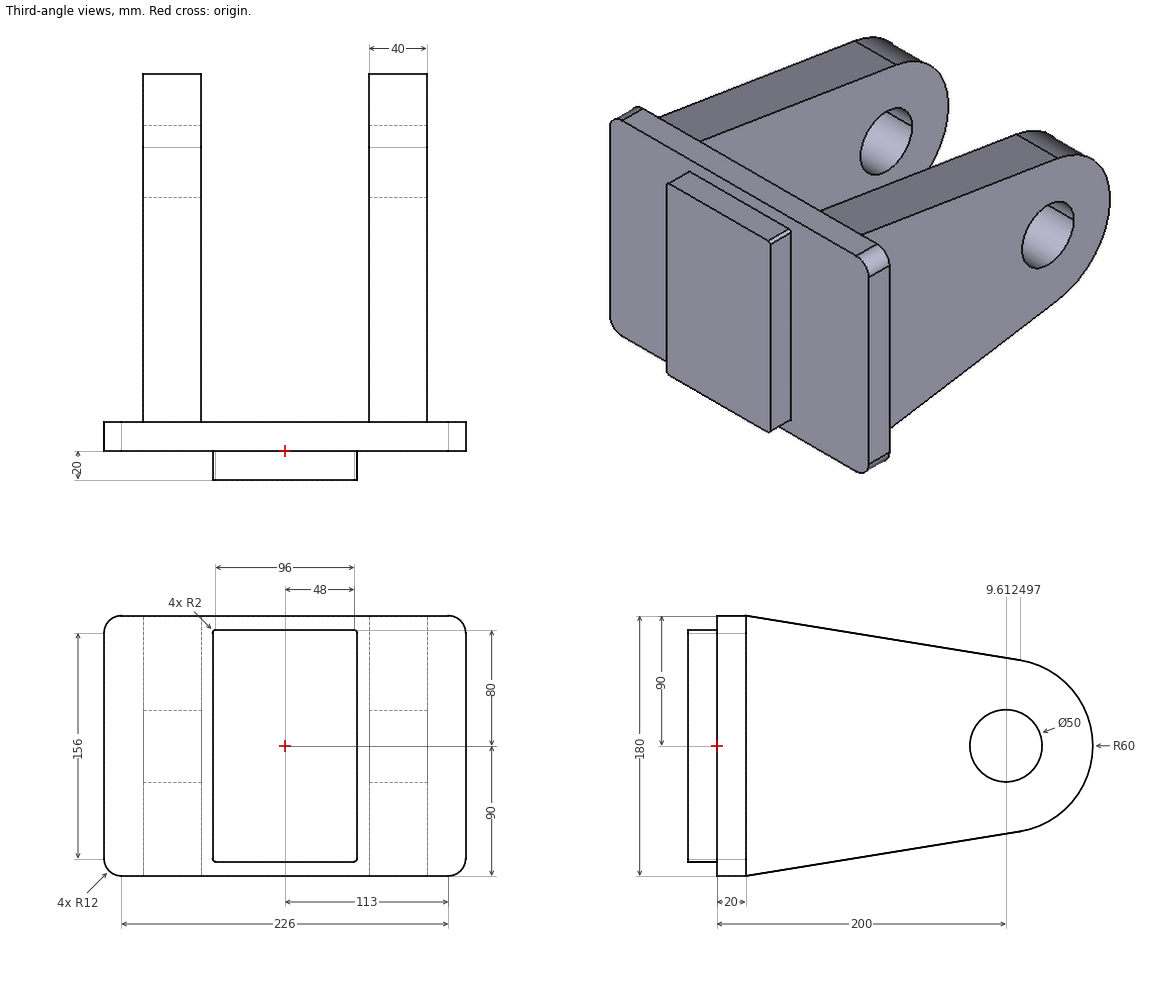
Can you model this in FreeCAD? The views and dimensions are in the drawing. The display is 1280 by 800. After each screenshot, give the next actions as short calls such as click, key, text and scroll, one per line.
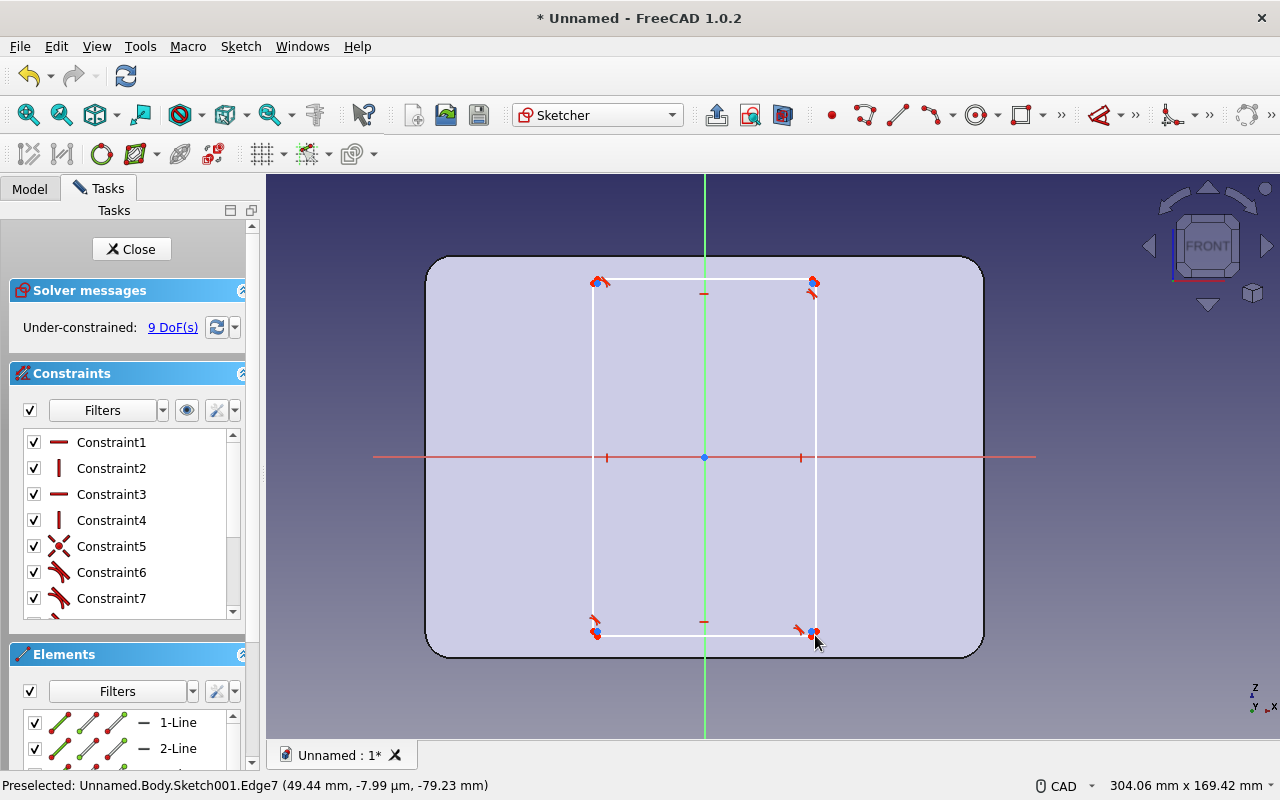
click(816, 562)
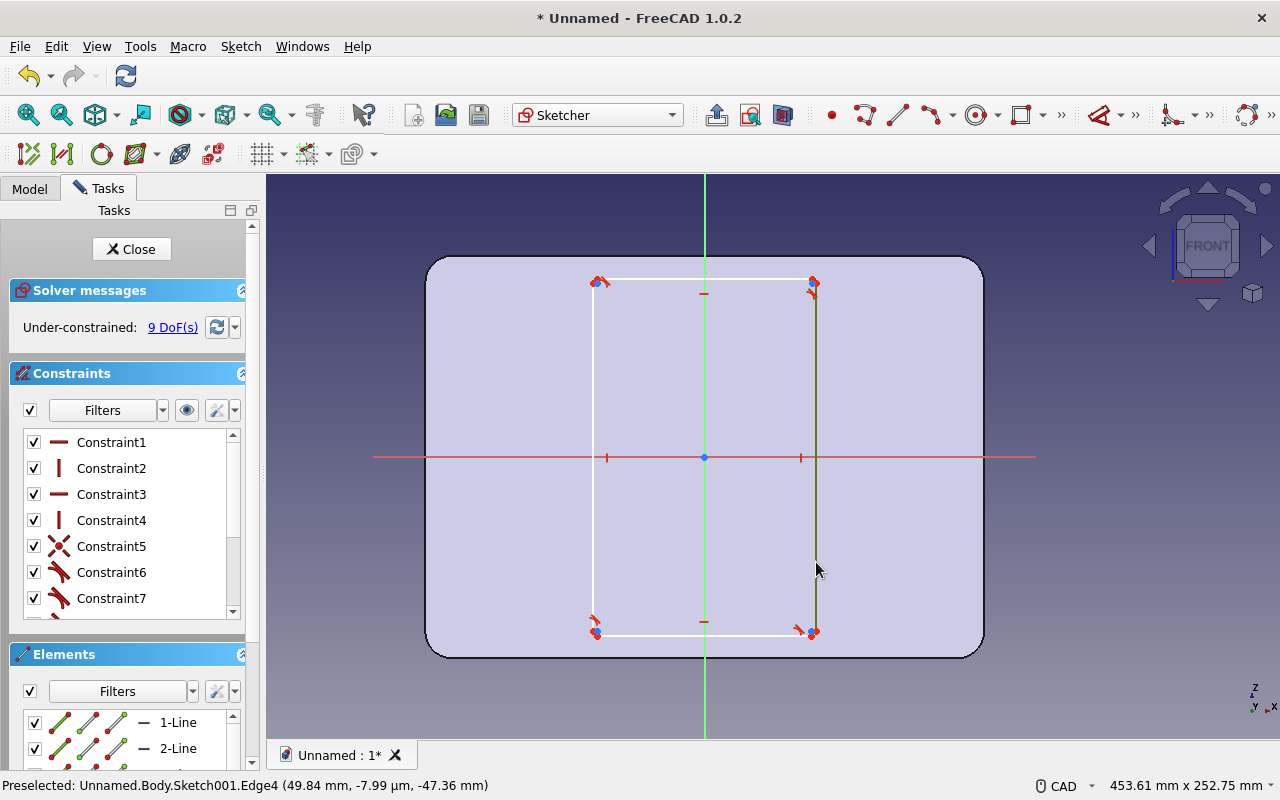
scroll(815, 281, up, 8)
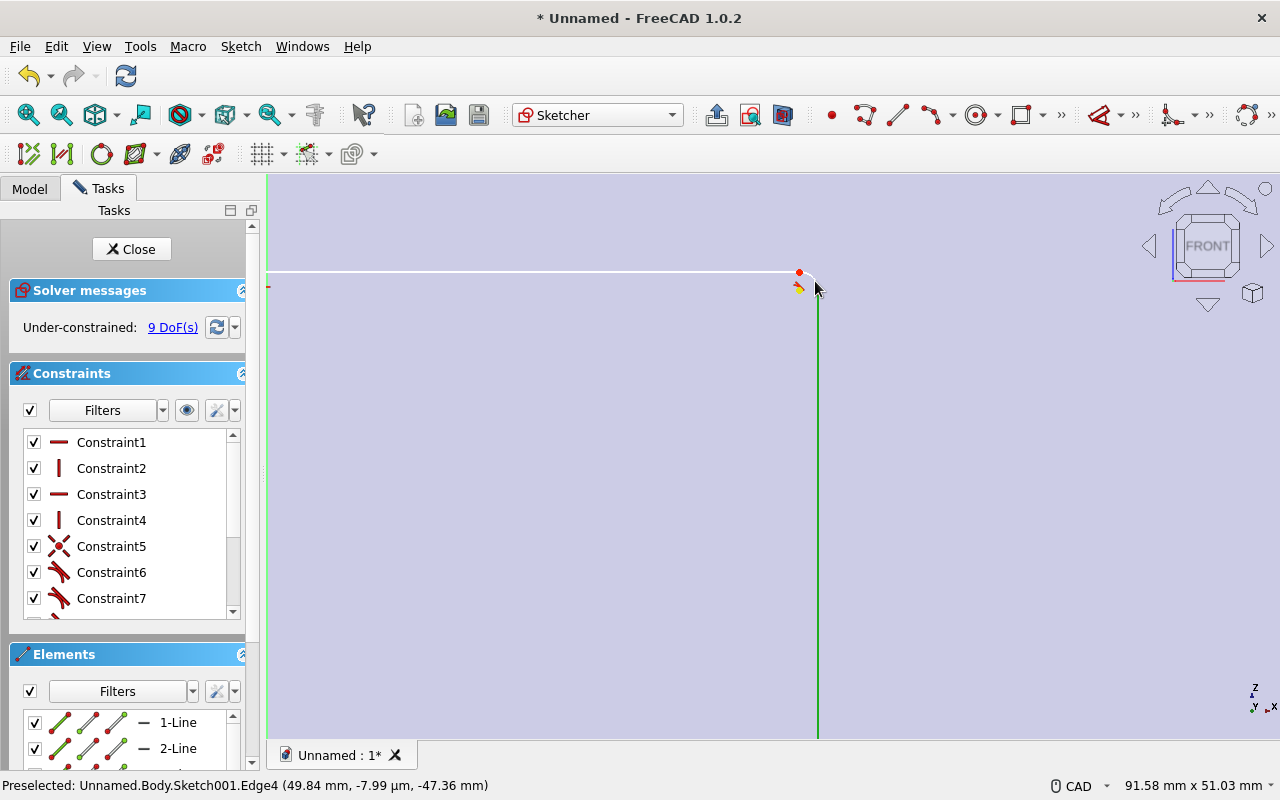
click(813, 278)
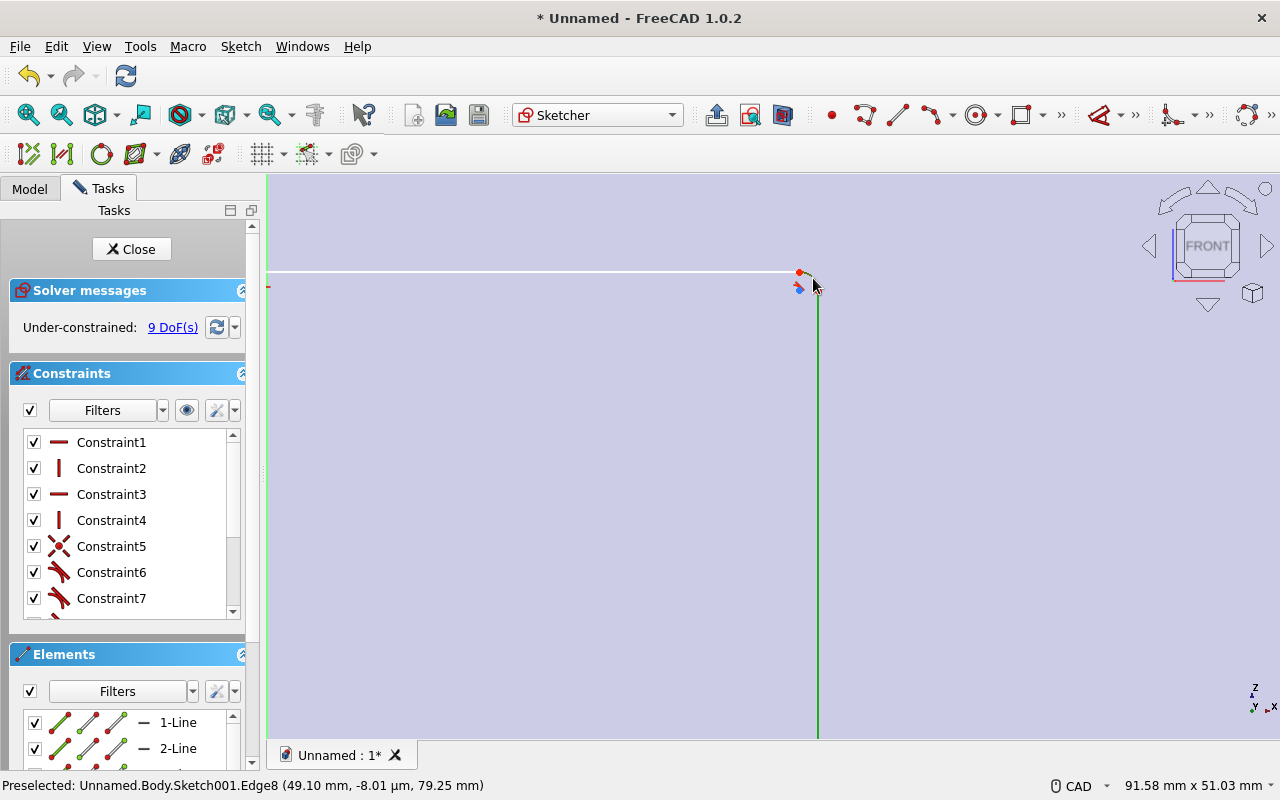
key(t)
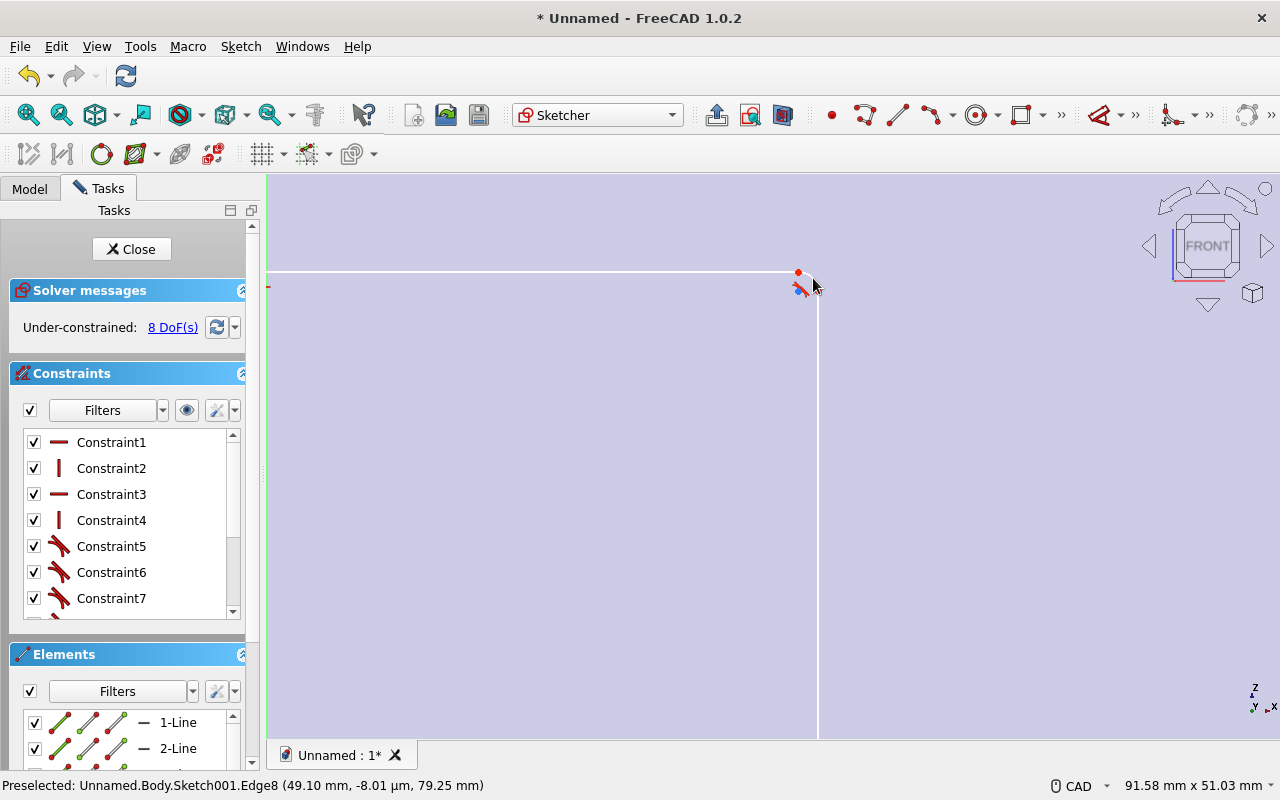
scroll(815, 280, down, 8)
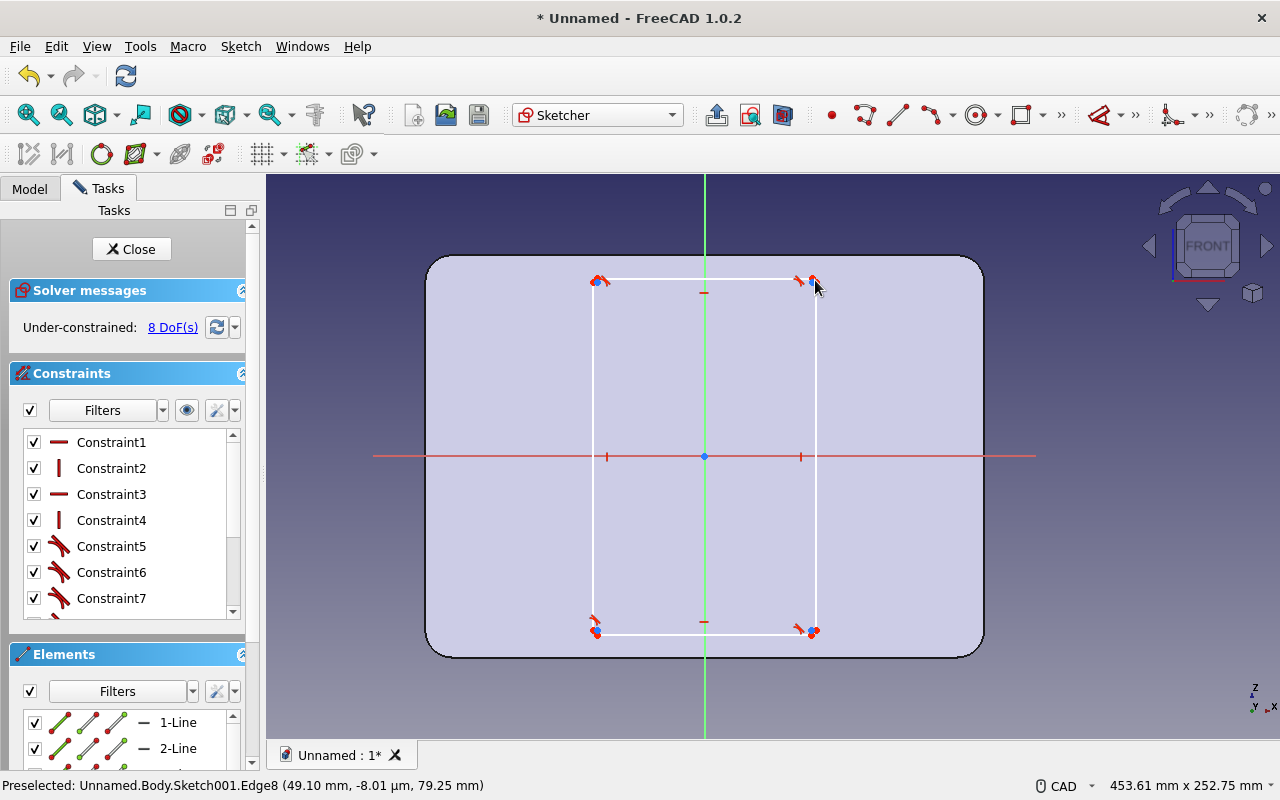
scroll(595, 279, up, 11)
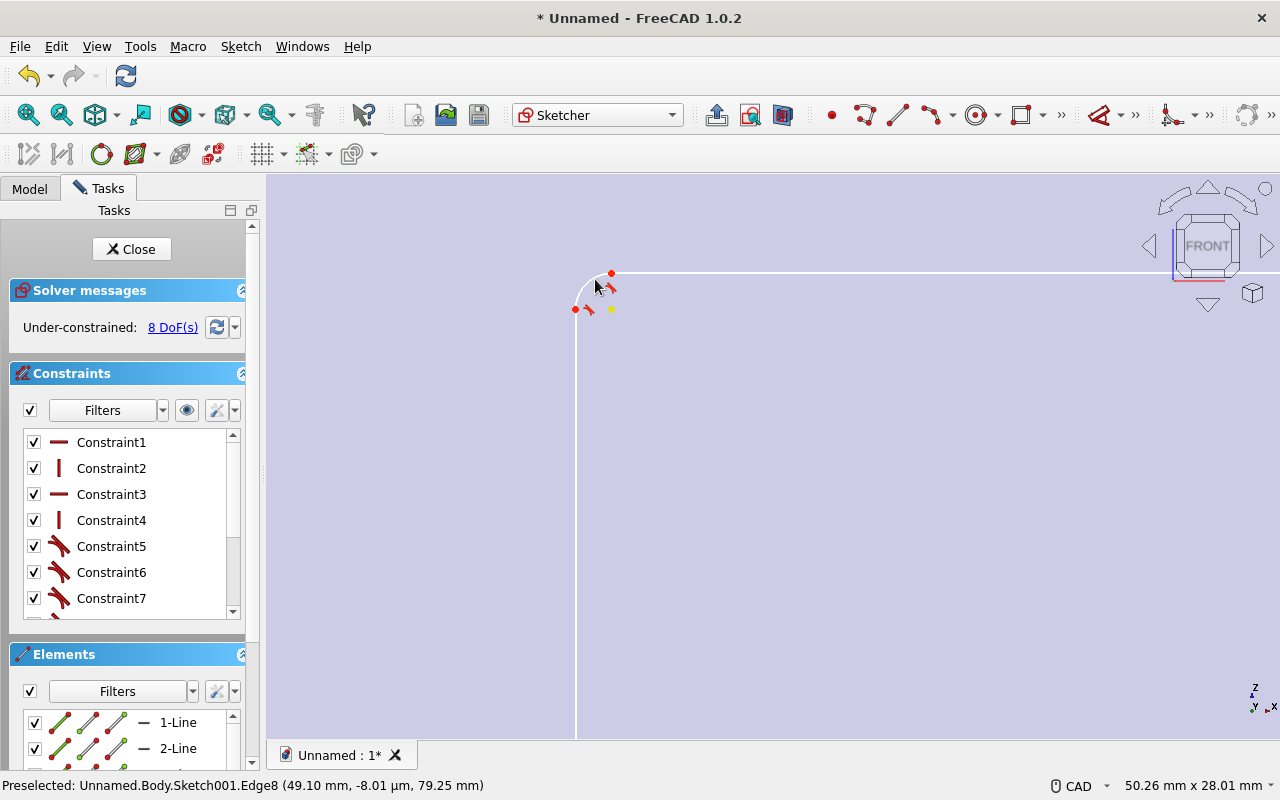
click(595, 277)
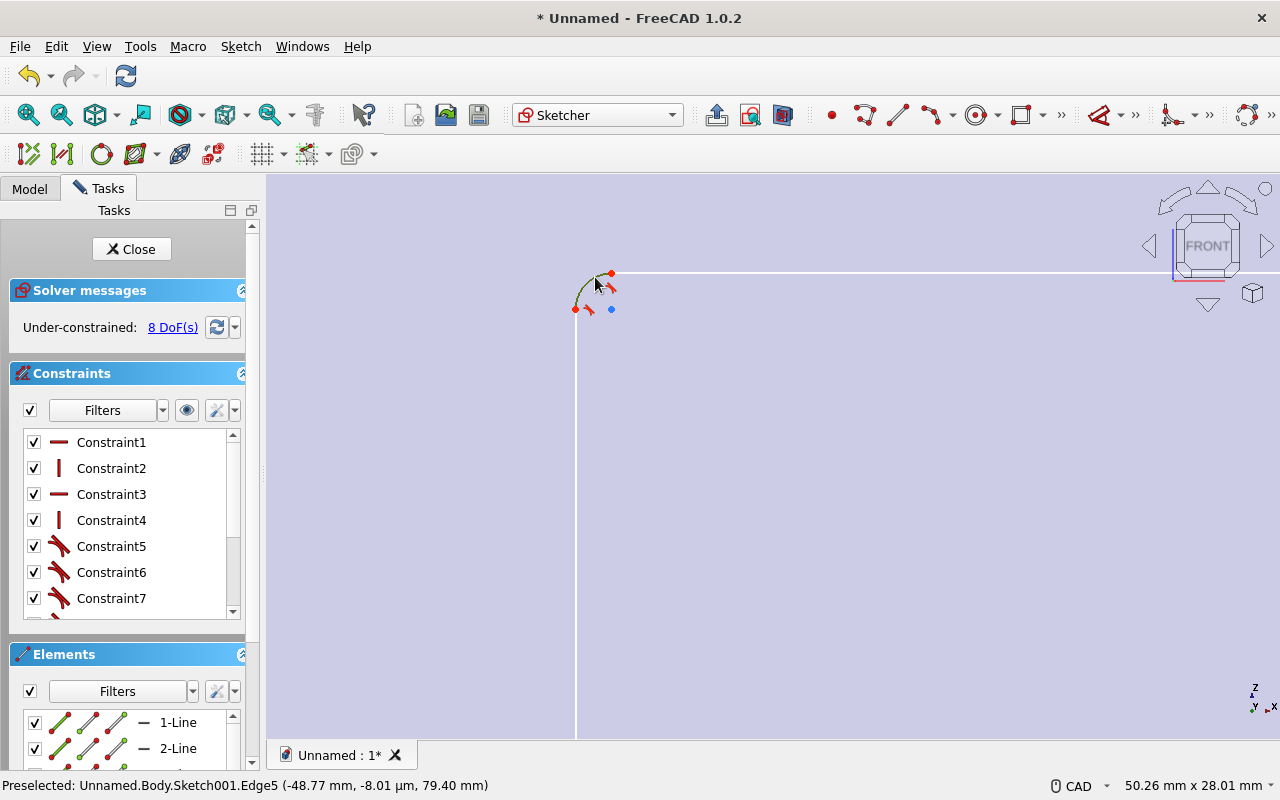
scroll(595, 279, down, 11)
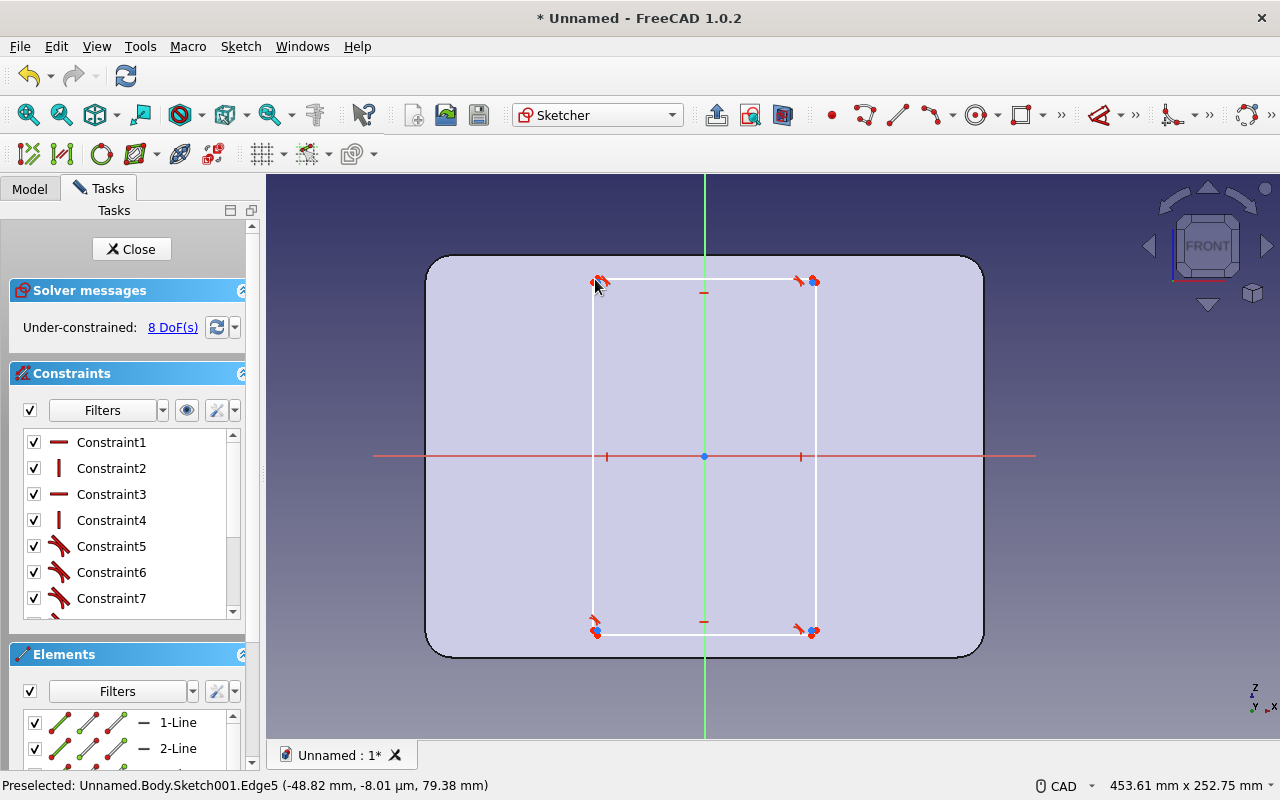
scroll(594, 633, up, 10)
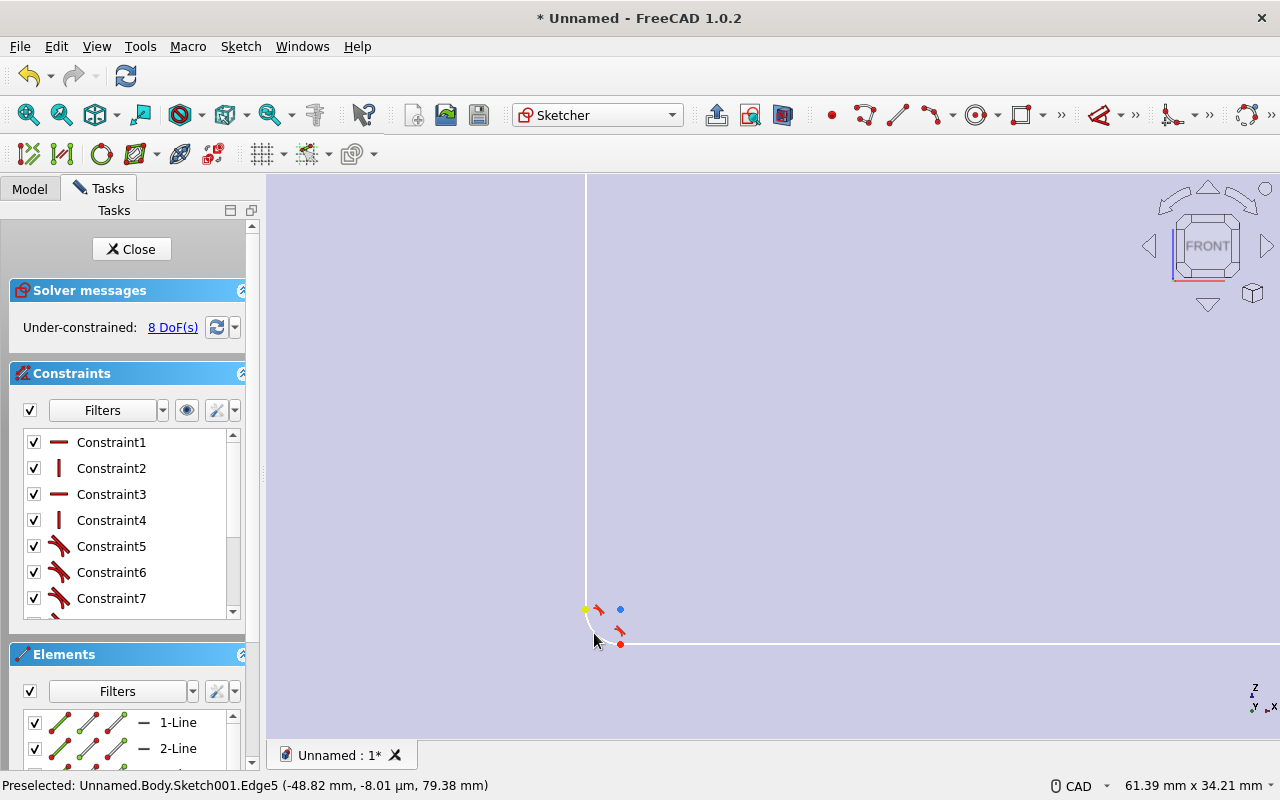
click(590, 625)